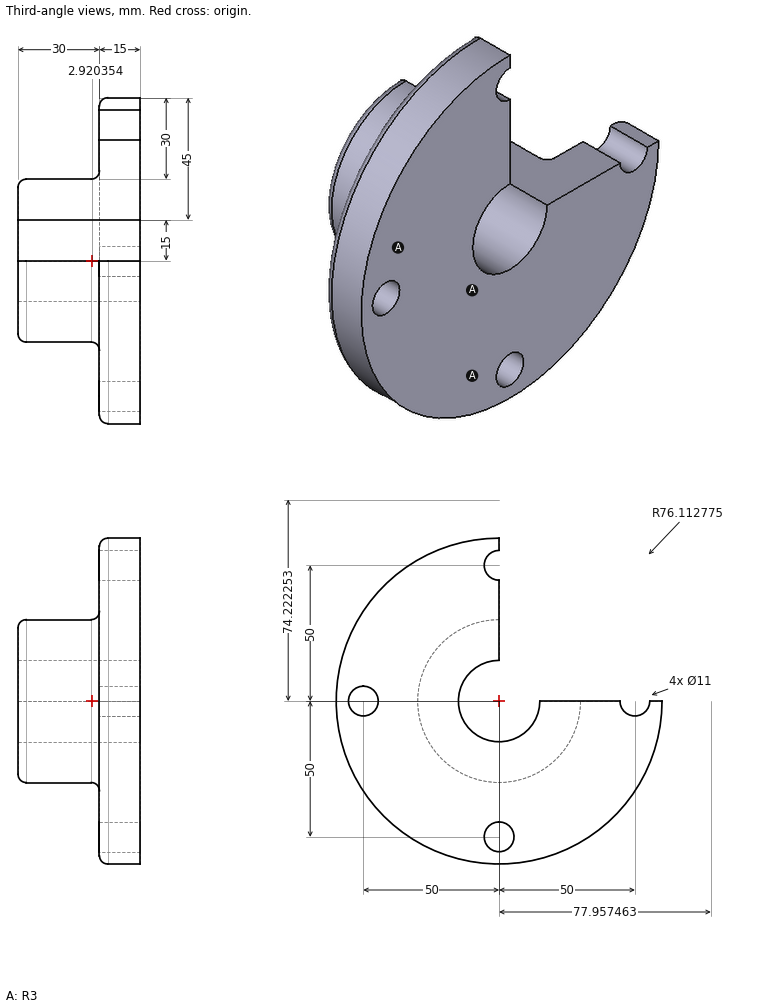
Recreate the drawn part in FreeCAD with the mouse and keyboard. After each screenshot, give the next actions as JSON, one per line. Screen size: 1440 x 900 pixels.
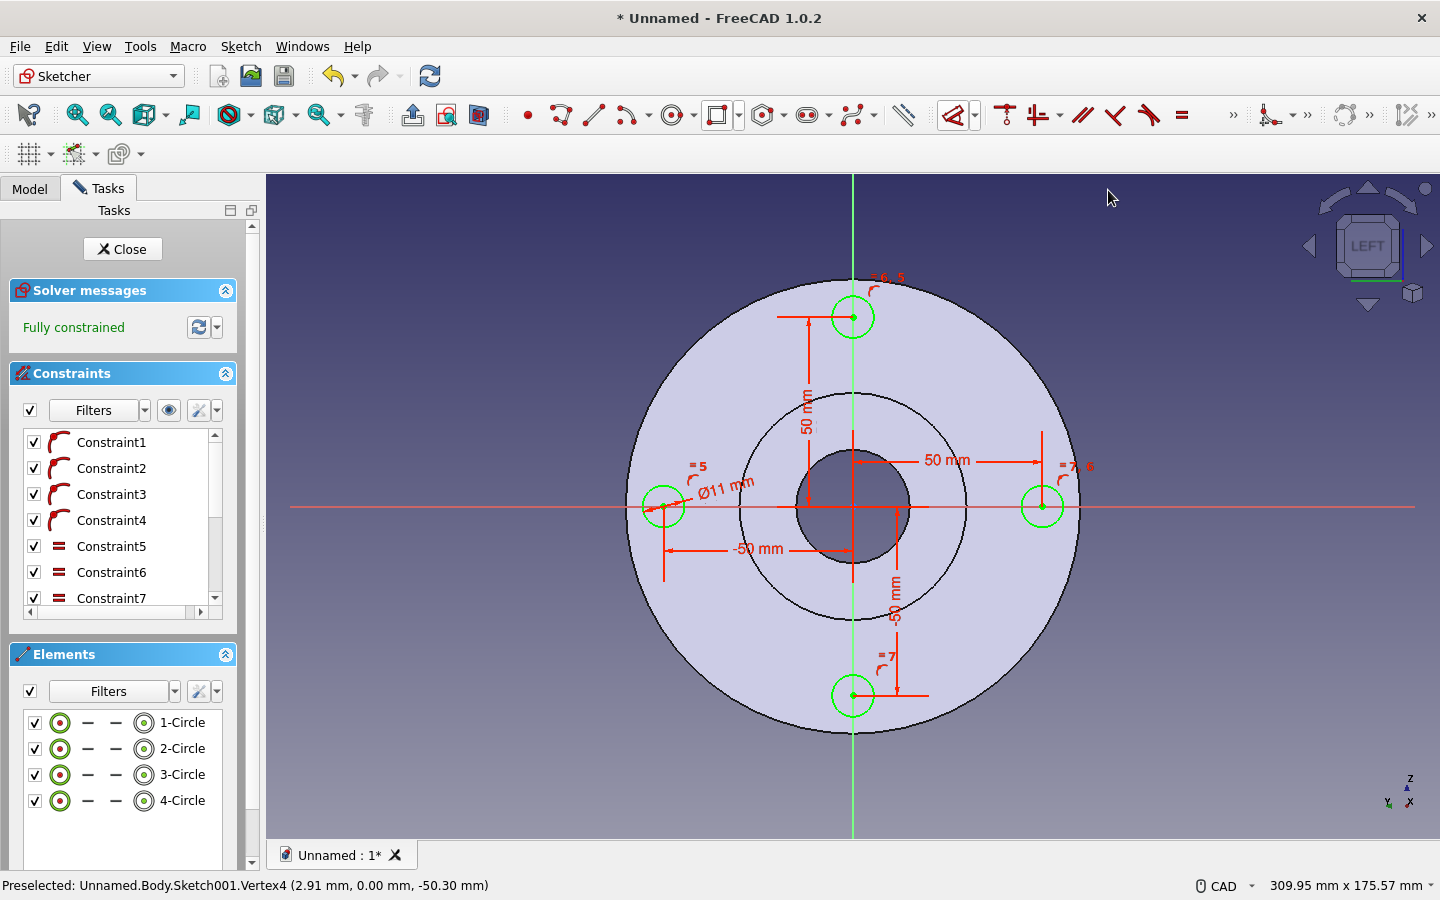
{"action": "left_click", "coordinate": [123, 249]}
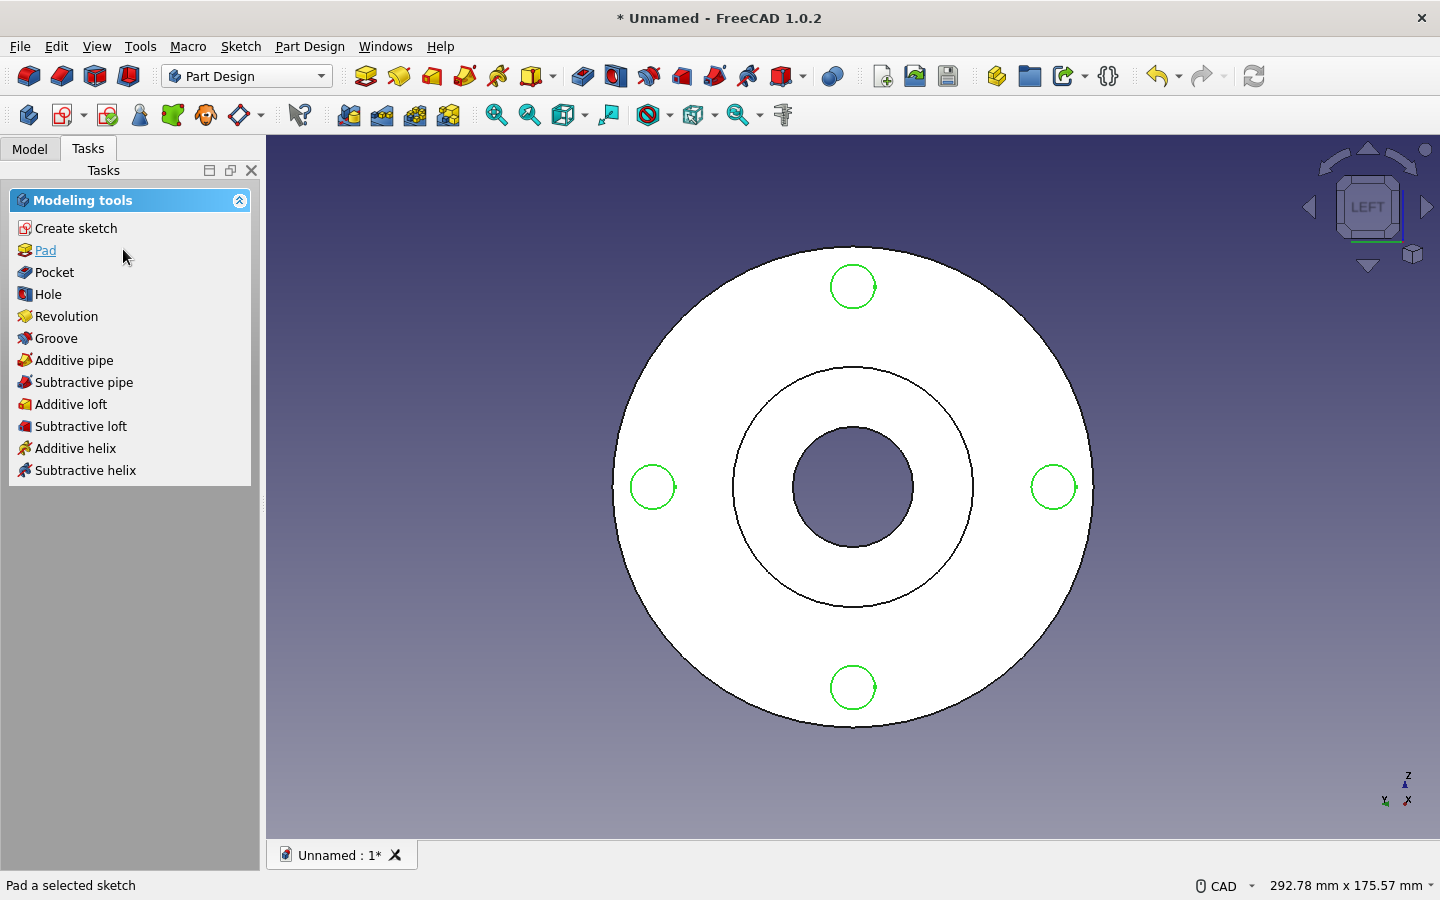
{"action": "left_click", "coordinate": [583, 76]}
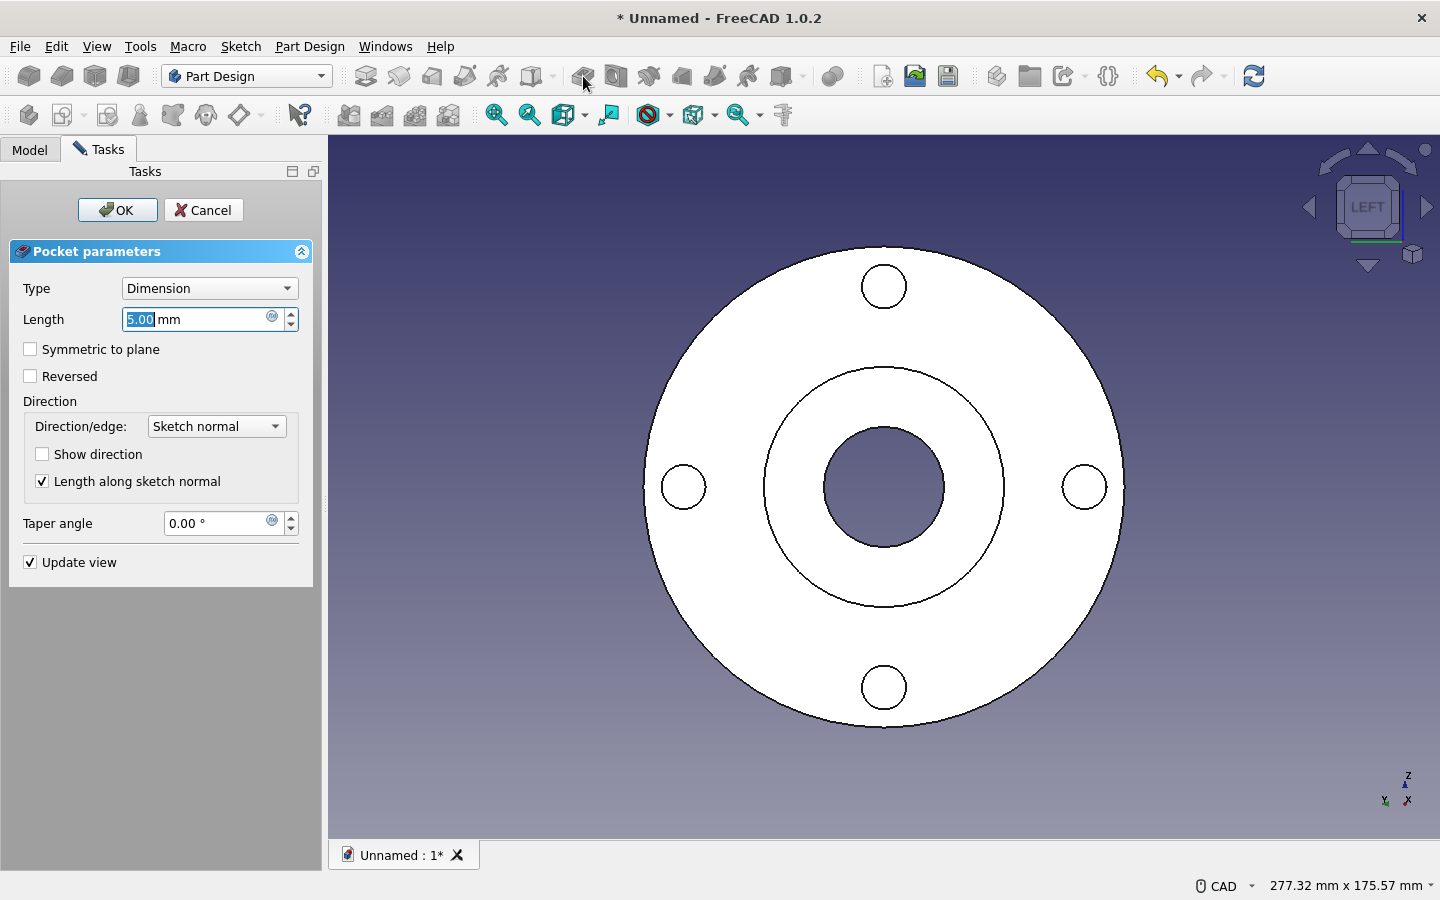
{"action": "left_click", "coordinate": [210, 288]}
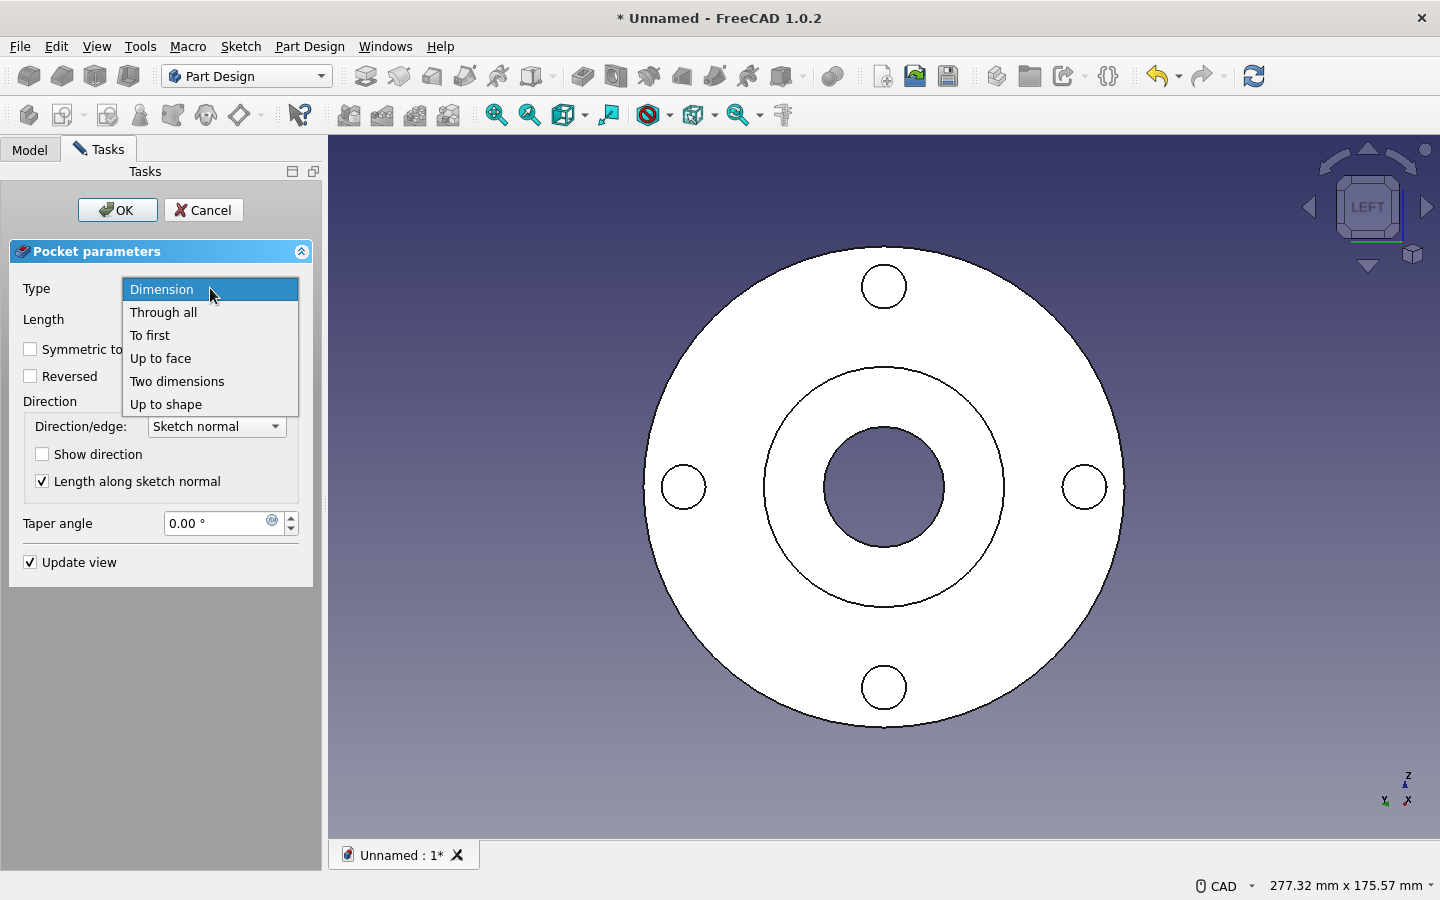
{"action": "left_click", "coordinate": [208, 312]}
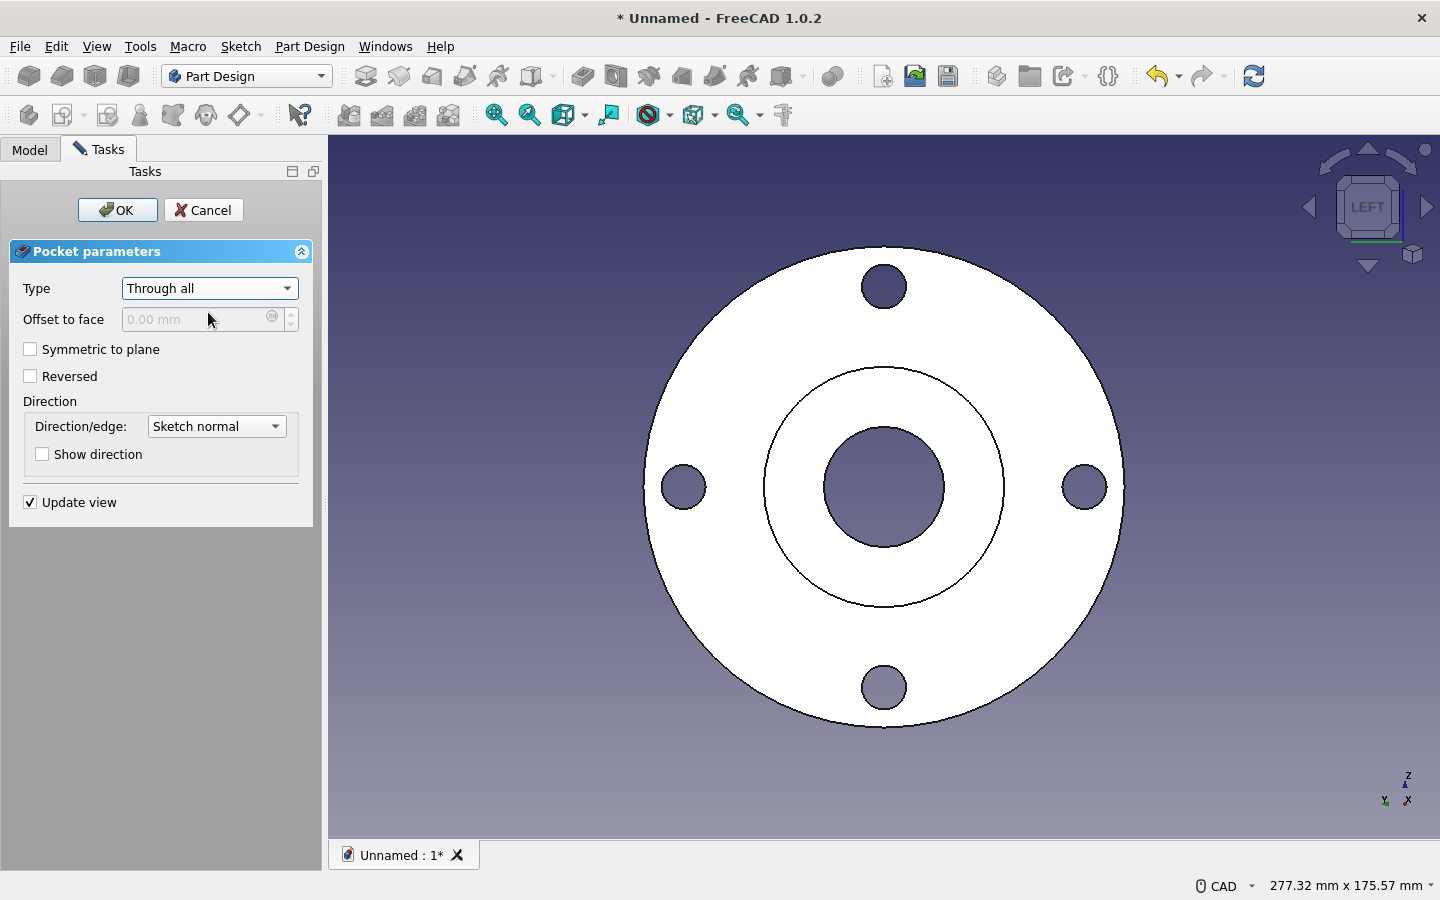
{"action": "left_click", "coordinate": [118, 210]}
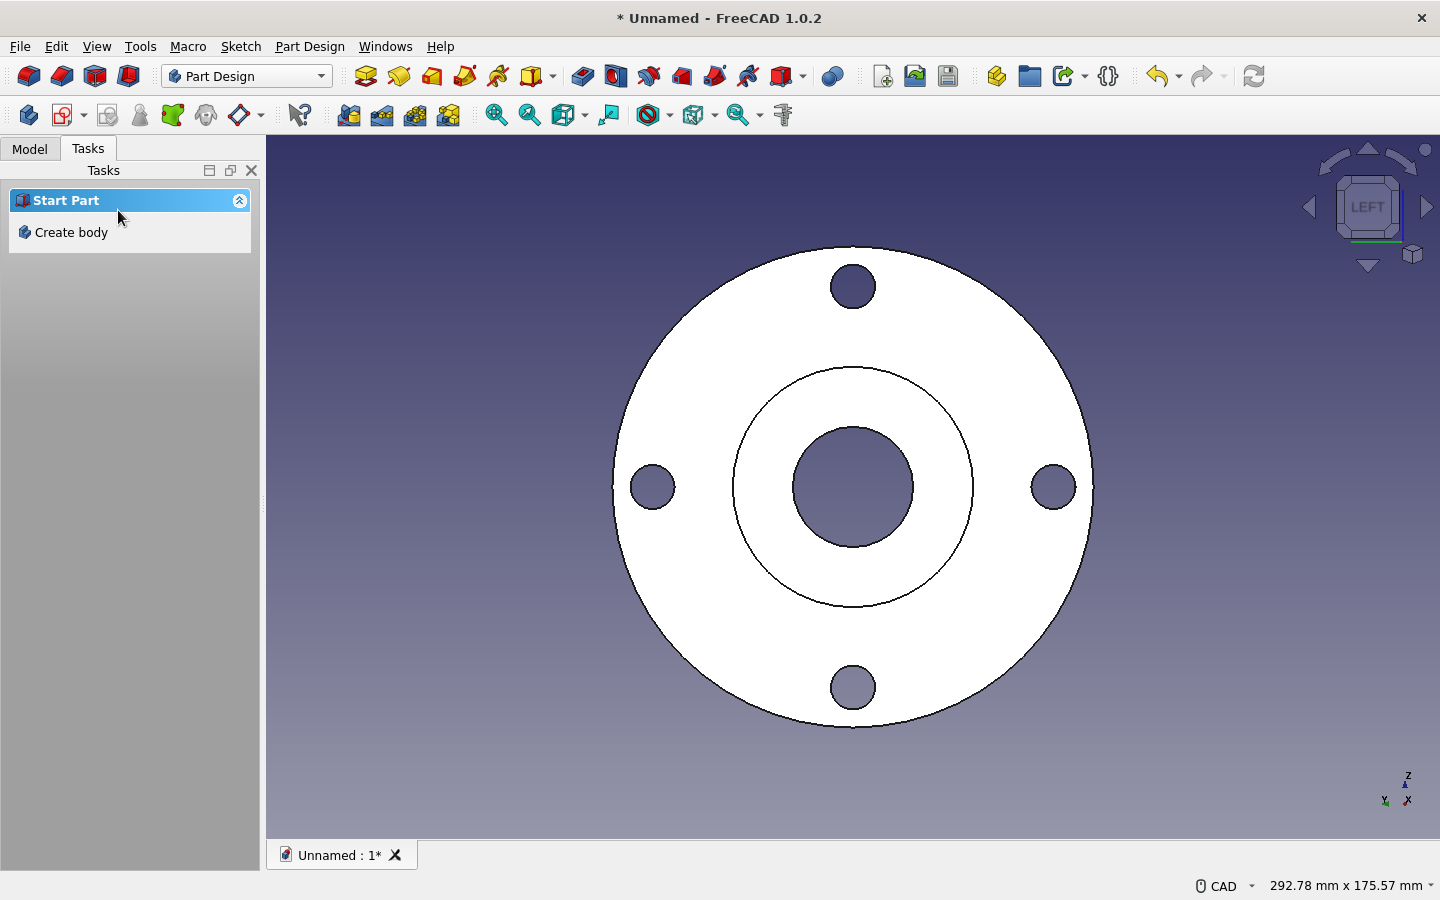
{"action": "left_click", "coordinate": [973, 486]}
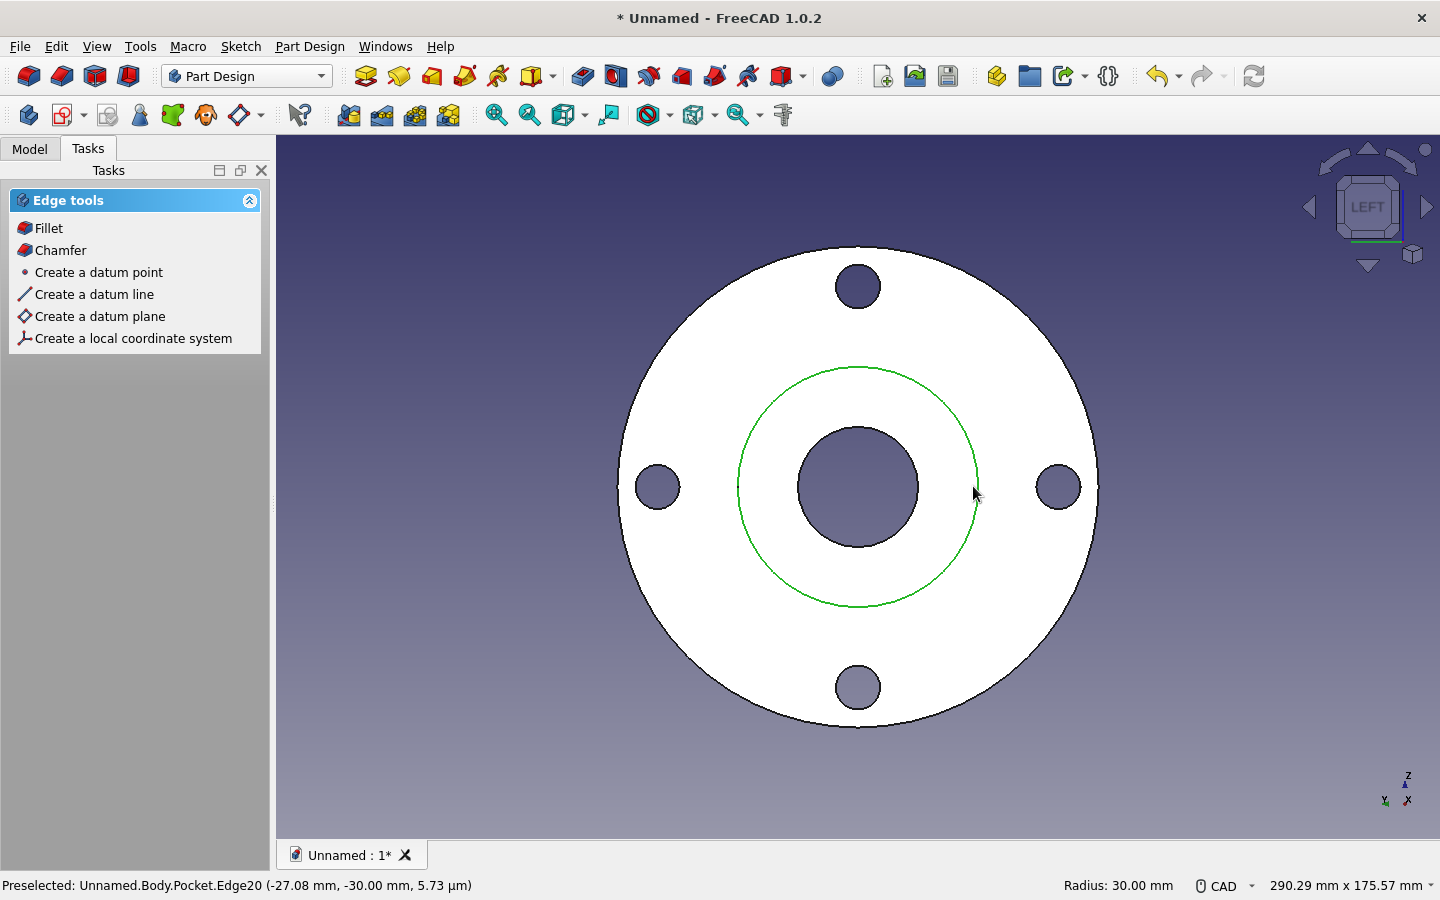
{"action": "left_click", "coordinate": [1099, 486], "text": "ctrl"}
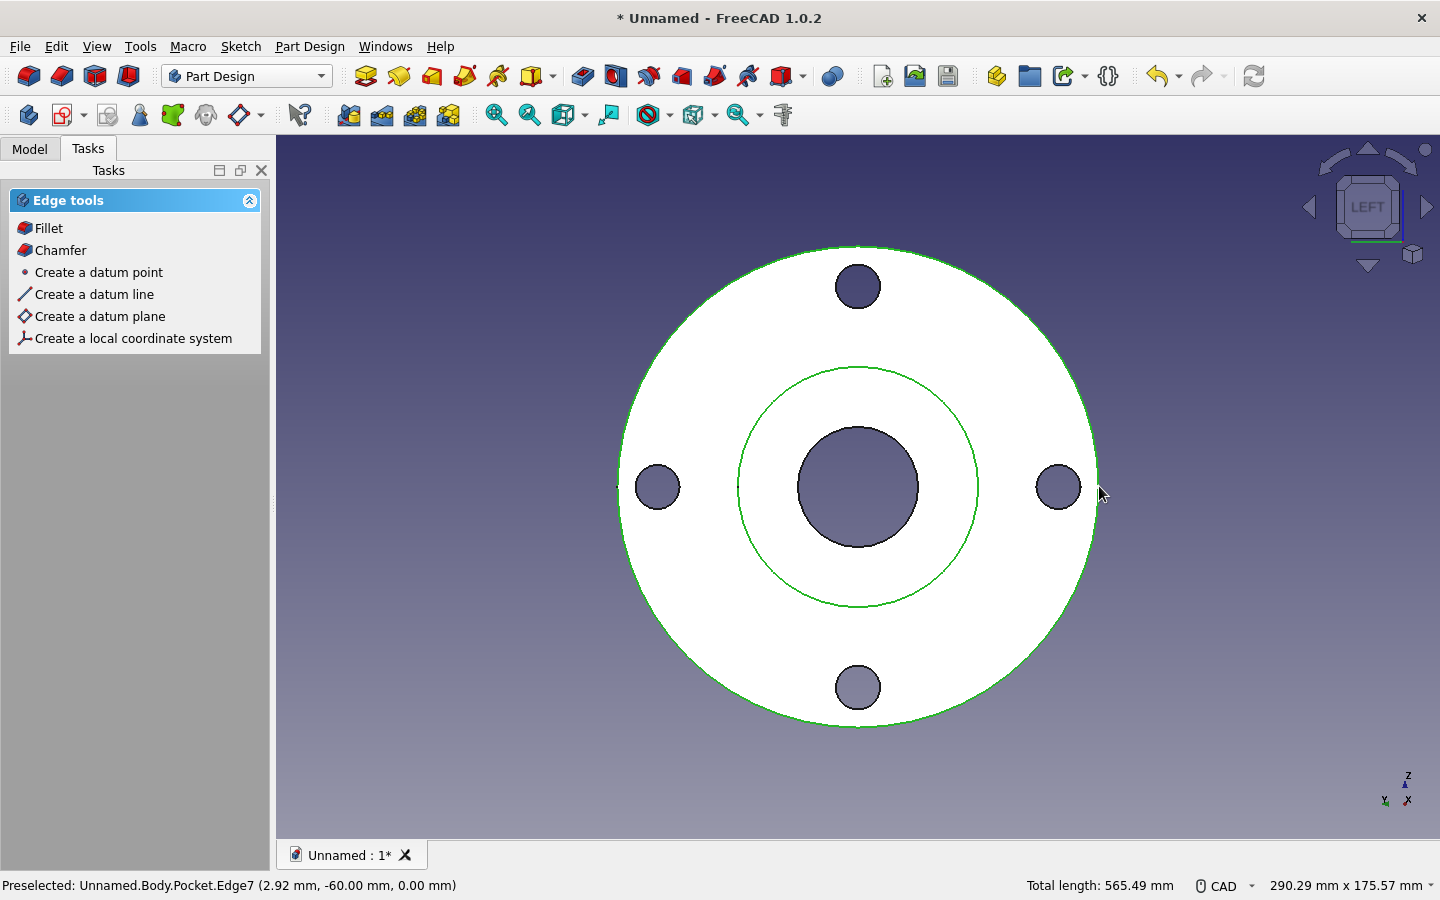
{"action": "key", "text": "0"}